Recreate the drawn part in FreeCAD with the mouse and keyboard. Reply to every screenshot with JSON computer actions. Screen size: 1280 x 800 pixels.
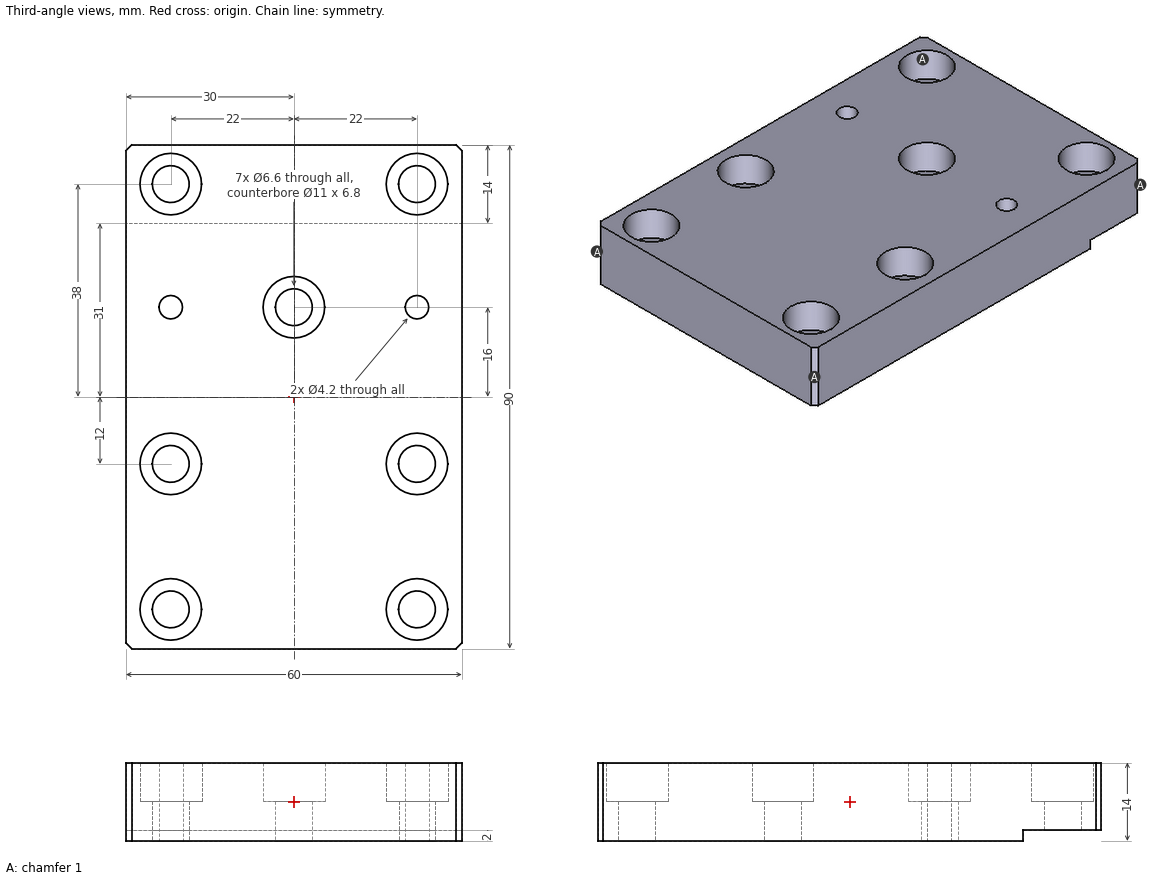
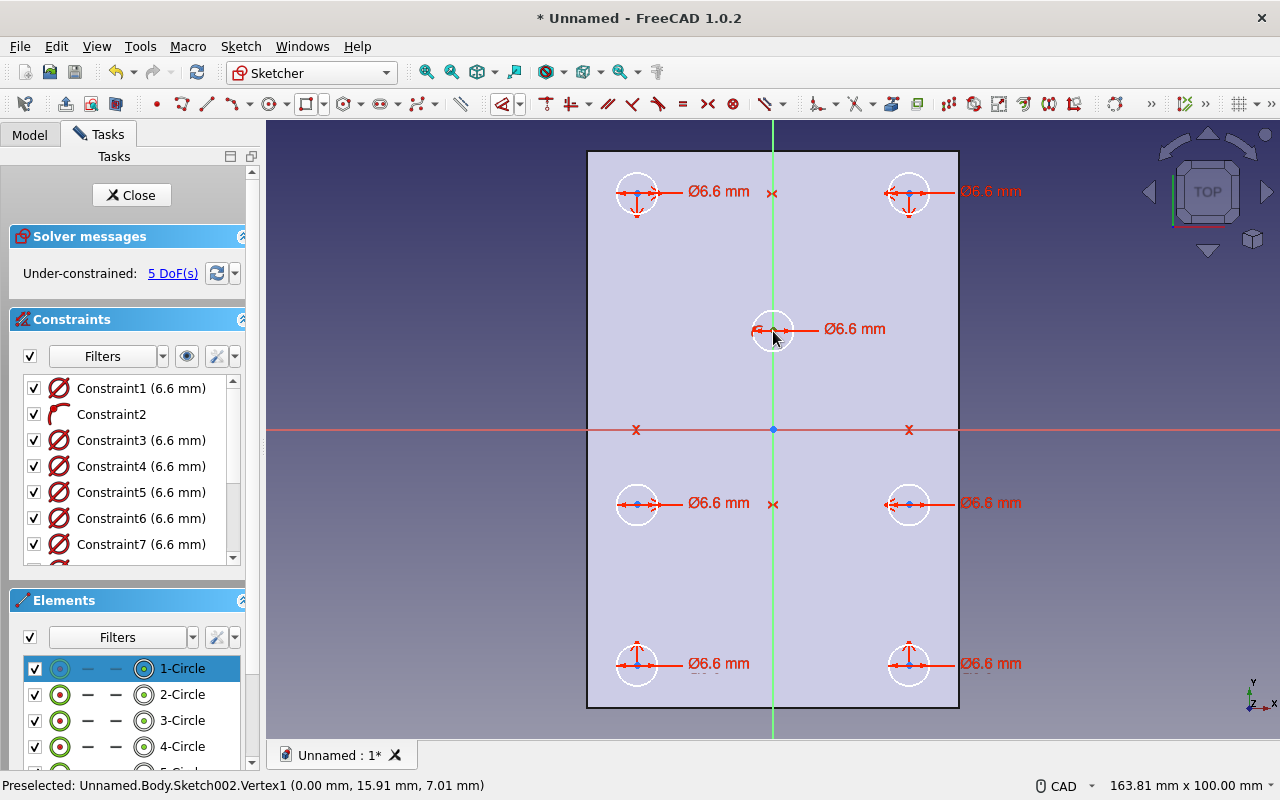
{"action": "key", "text": "i"}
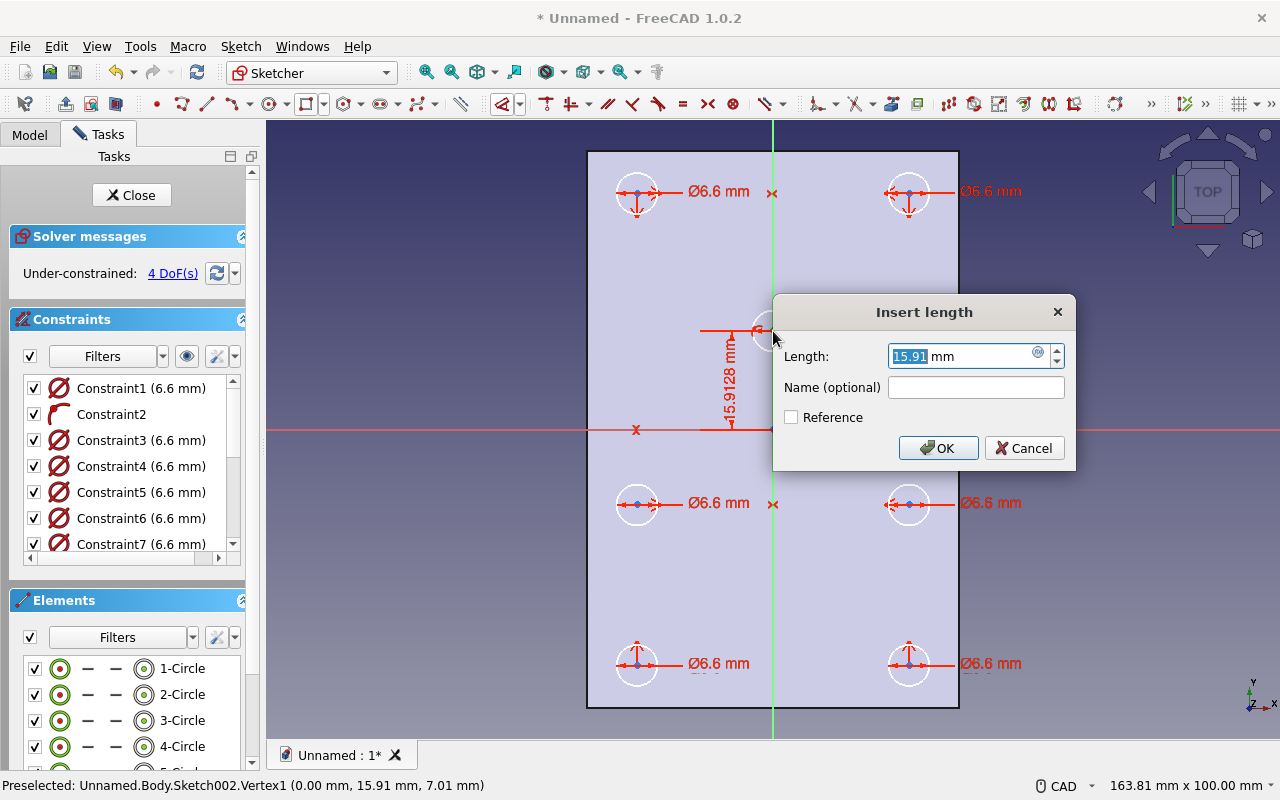
{"action": "type", "text": "16"}
{"action": "key", "text": "Return"}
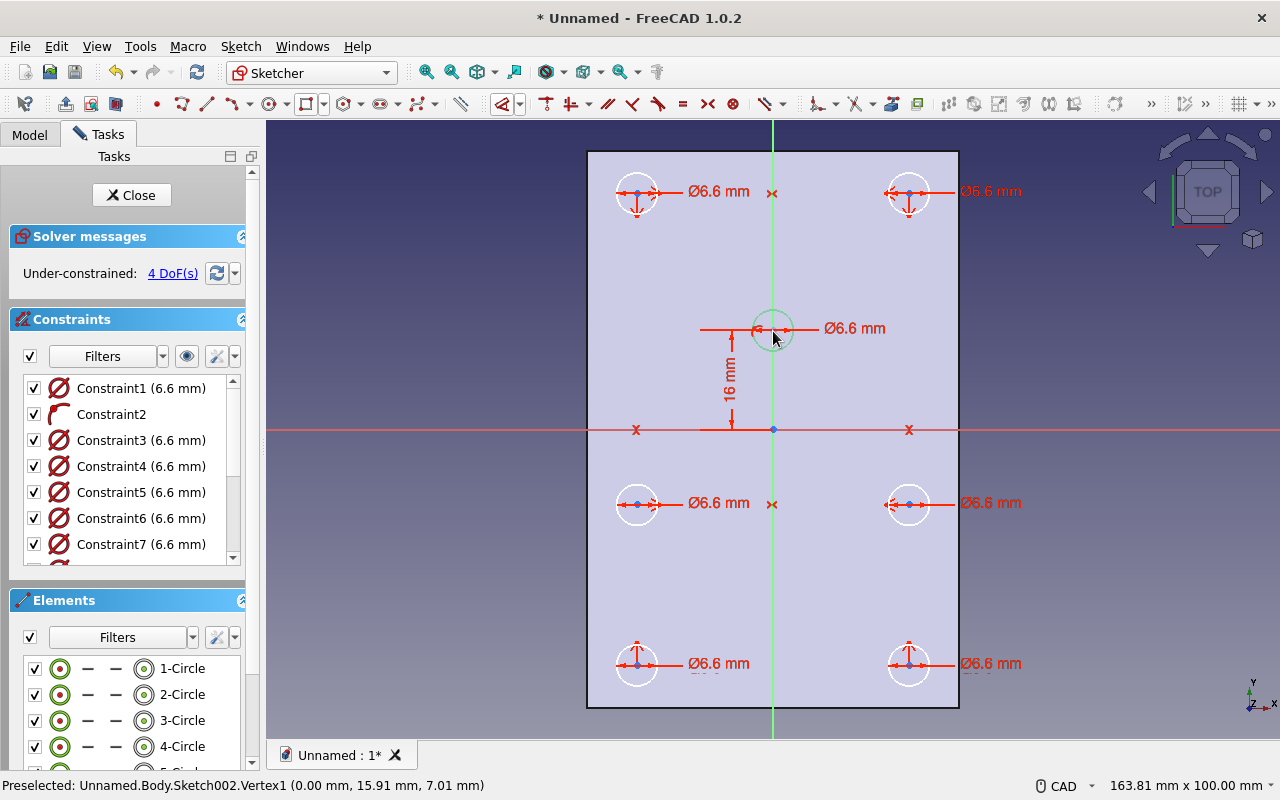
{"action": "left_click", "coordinate": [637, 193]}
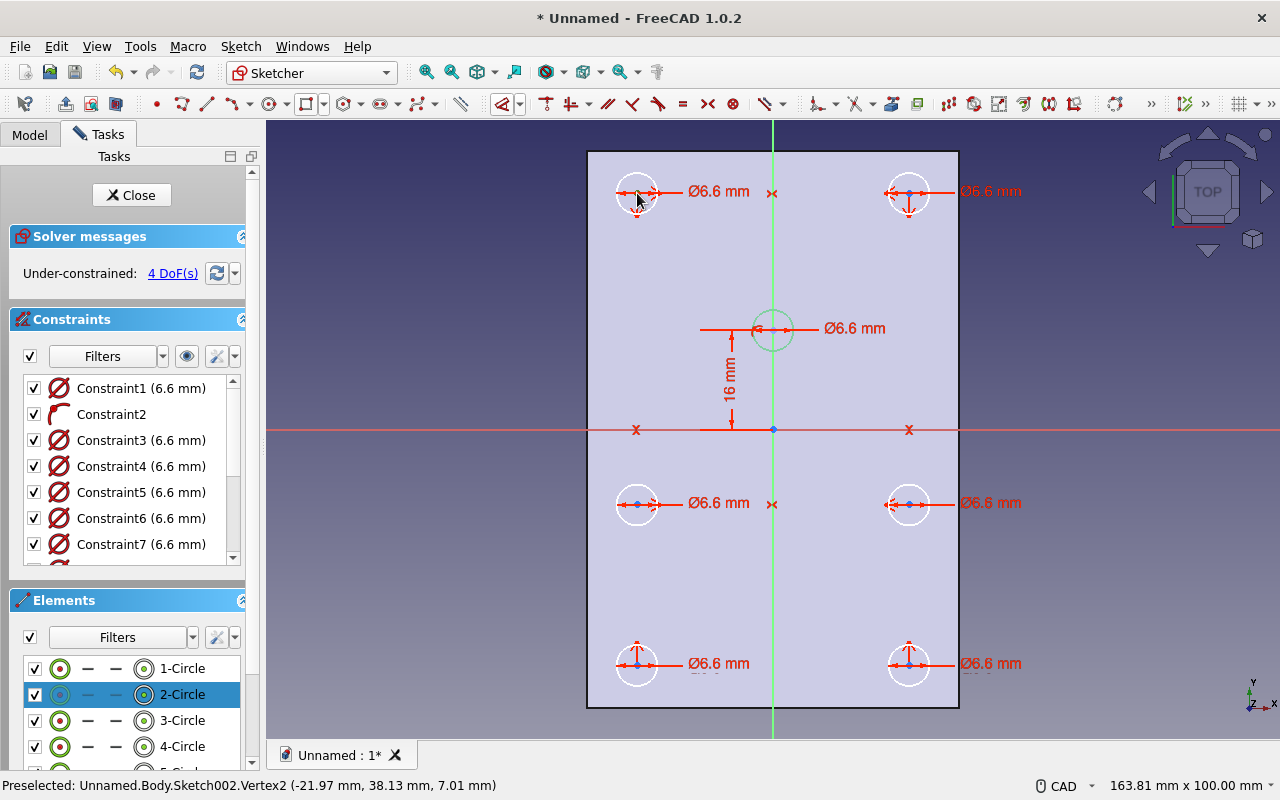
{"action": "left_click", "coordinate": [520, 104]}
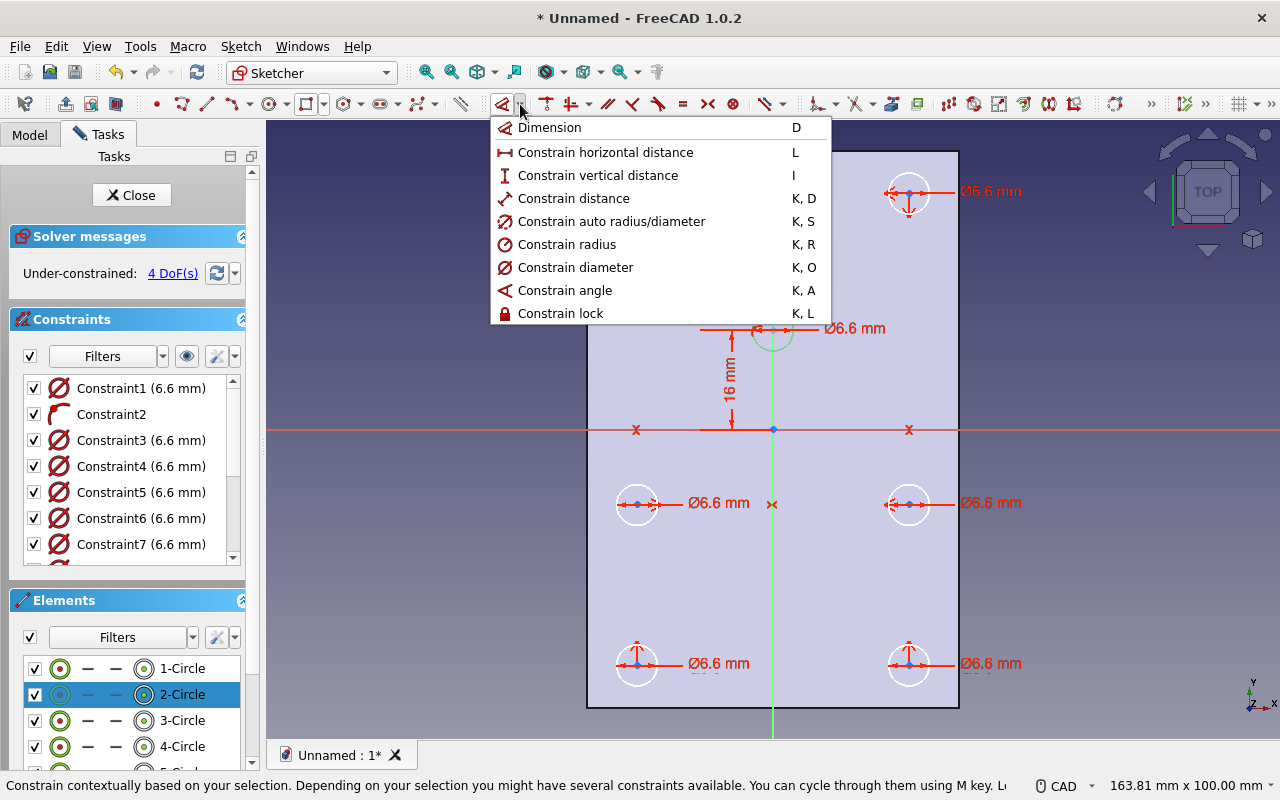
{"action": "left_click", "coordinate": [661, 152]}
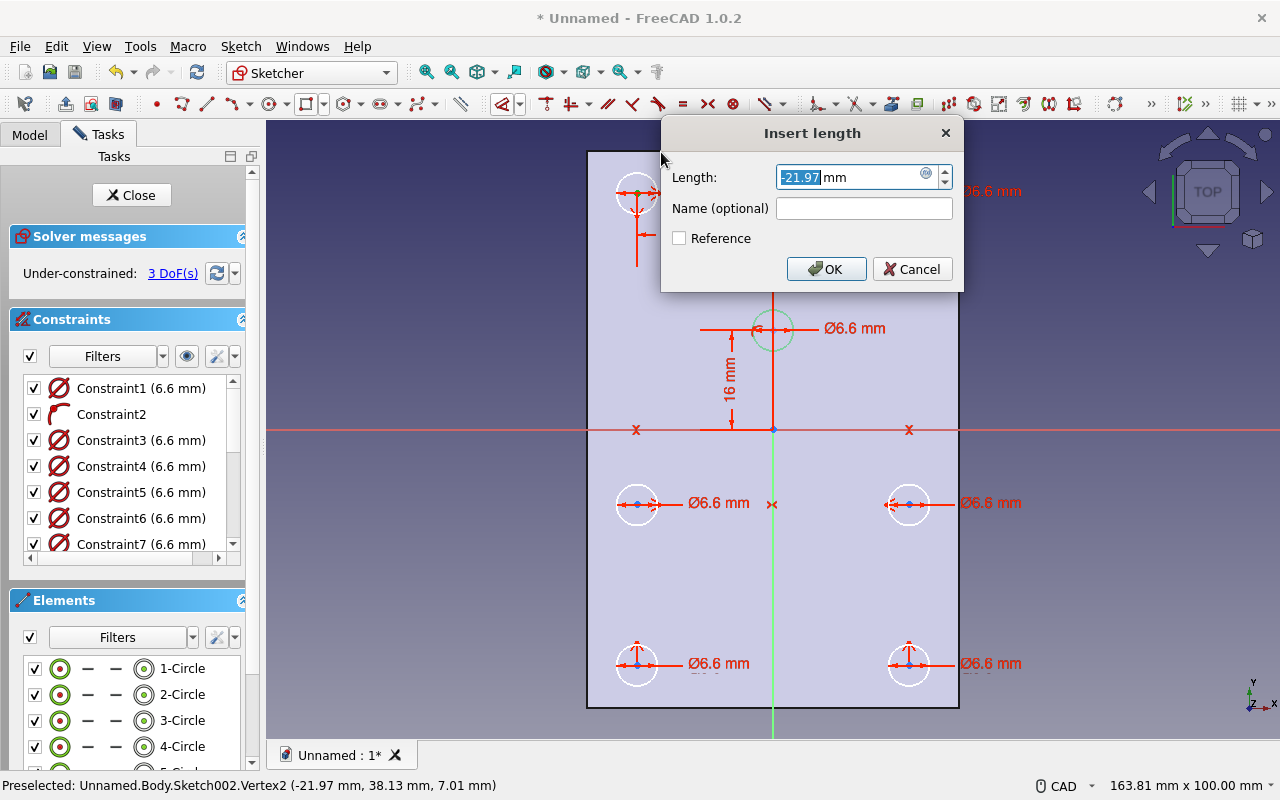
{"action": "type", "text": "-22"}
{"action": "key", "text": "Return"}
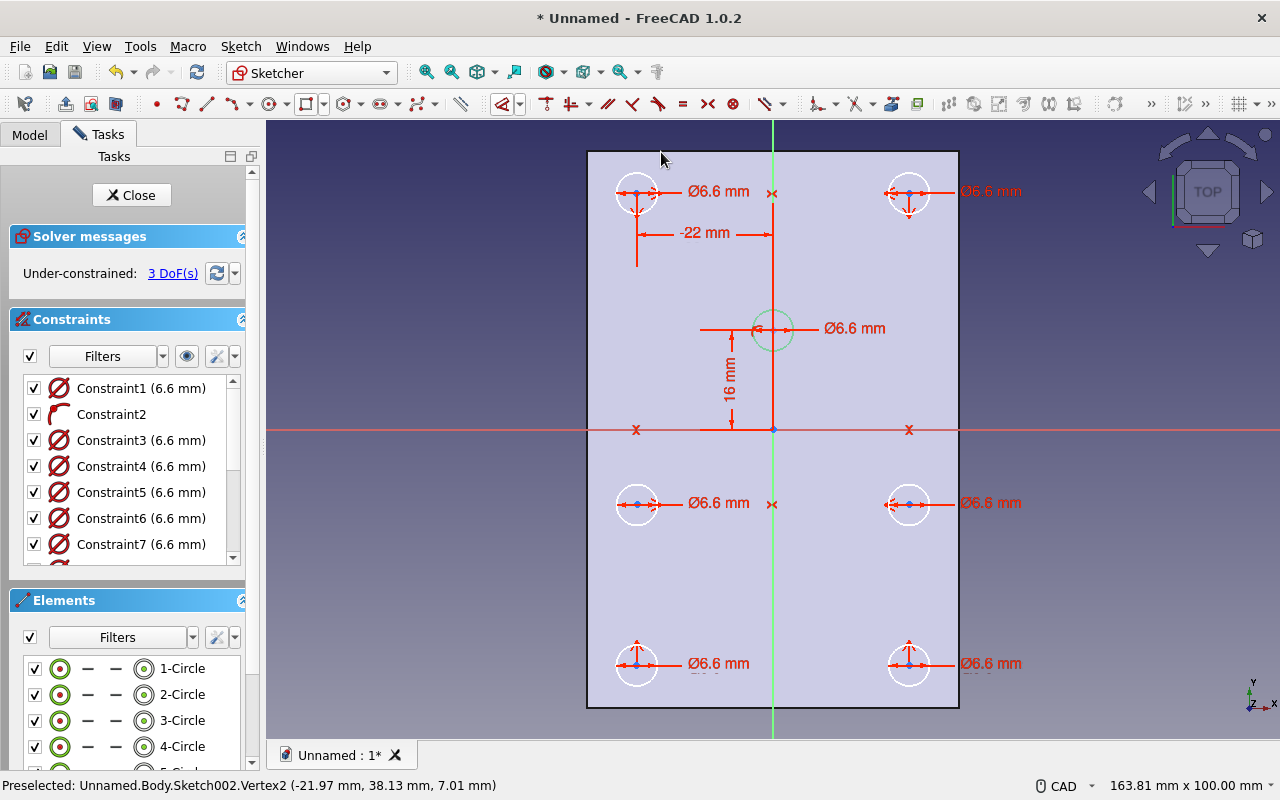
{"action": "left_click", "coordinate": [637, 193]}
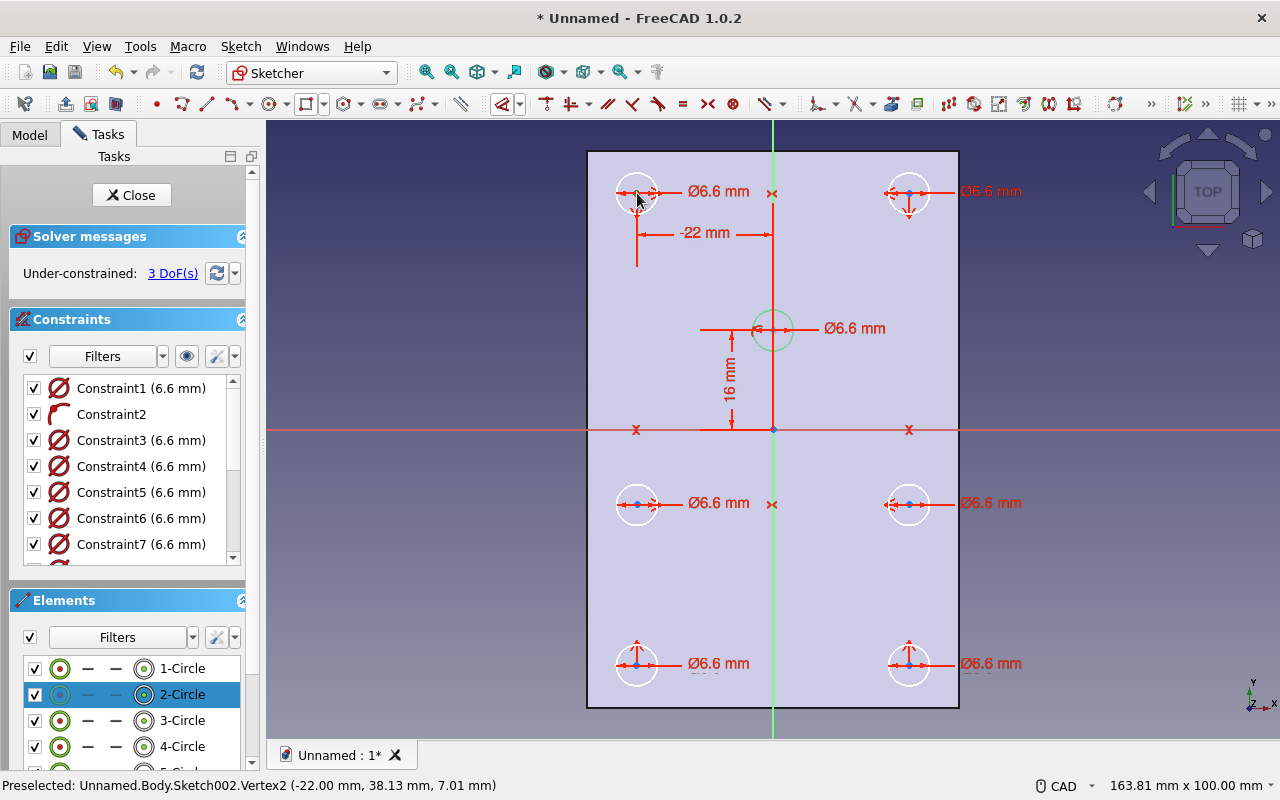
{"action": "left_click", "coordinate": [520, 104]}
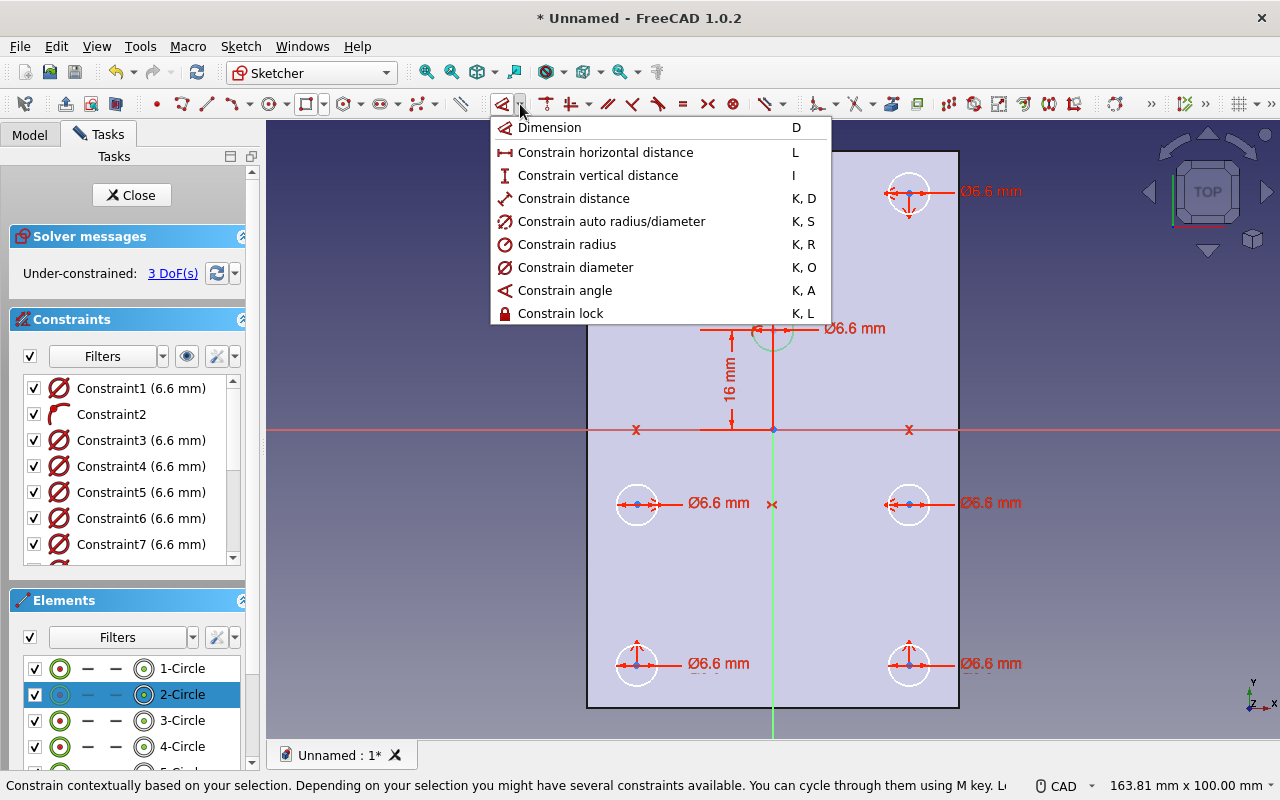
{"action": "left_click", "coordinate": [661, 176]}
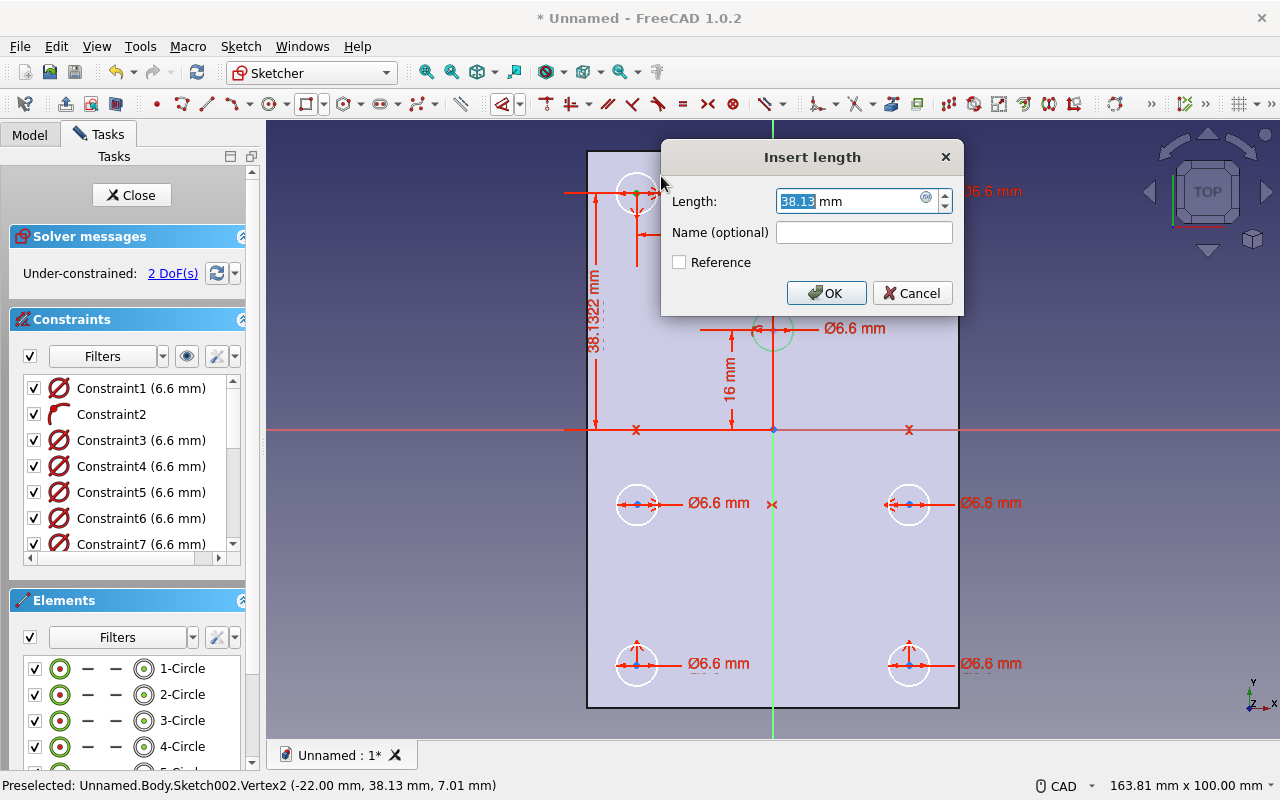
{"action": "type", "text": "38"}
{"action": "key", "text": "Return"}